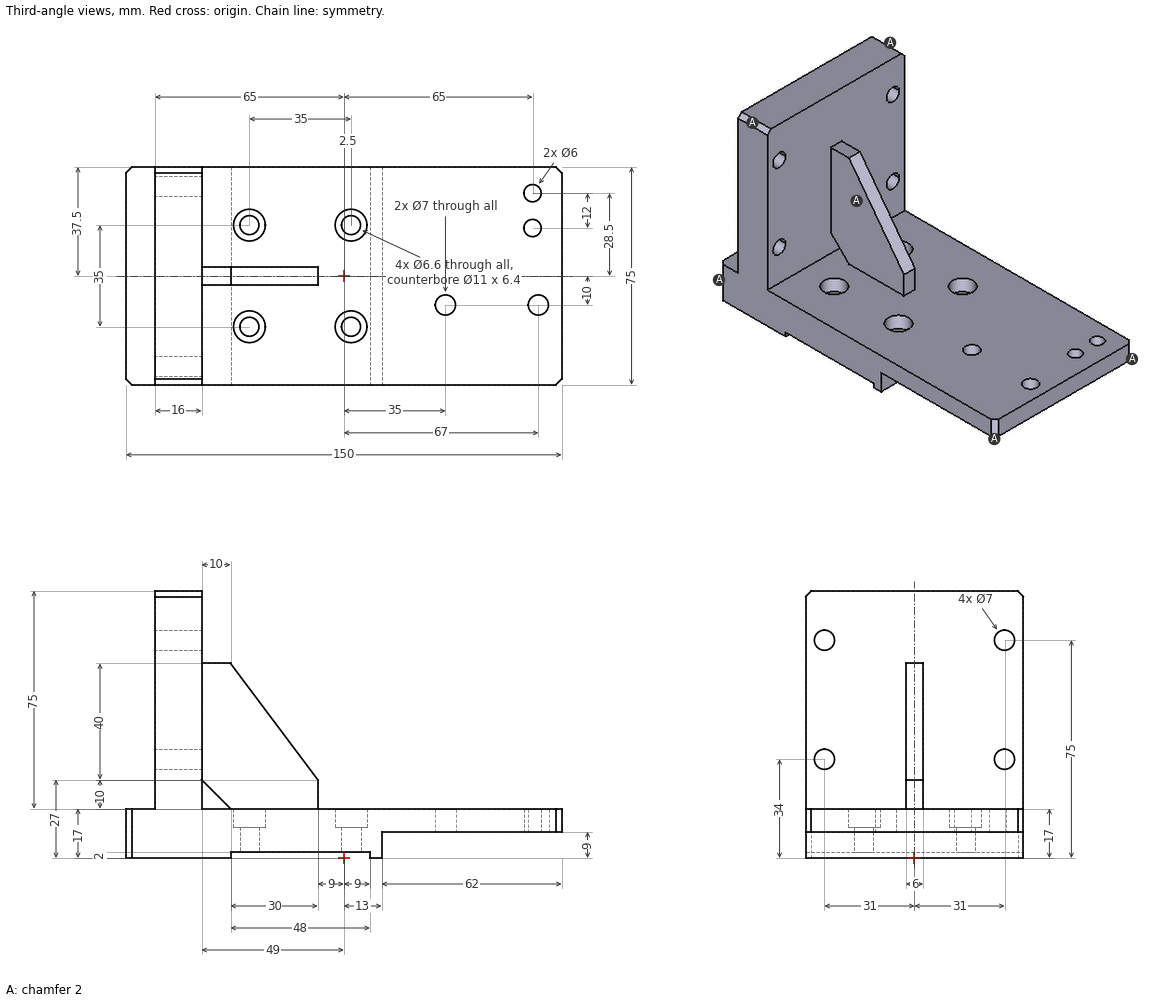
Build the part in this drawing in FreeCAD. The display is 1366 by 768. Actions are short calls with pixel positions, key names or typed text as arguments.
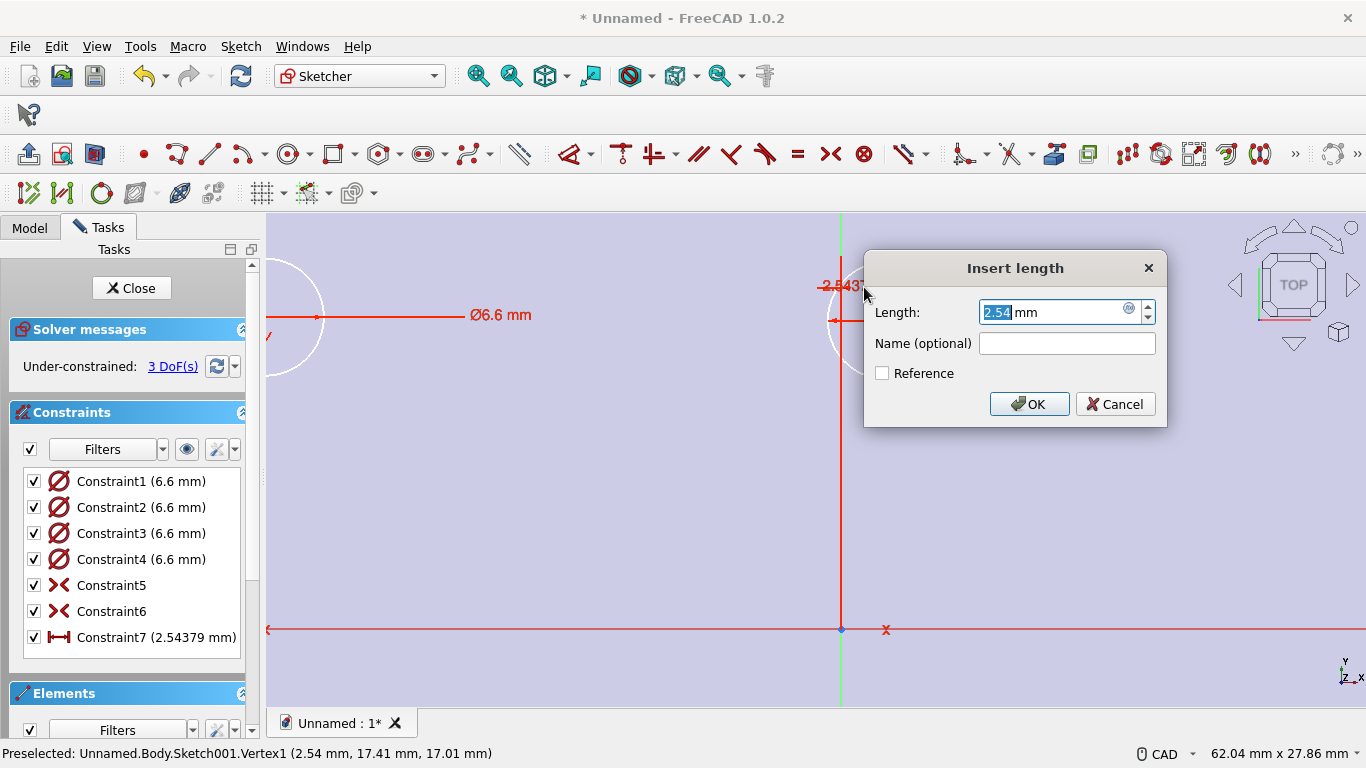
text(2.5)
key(Return)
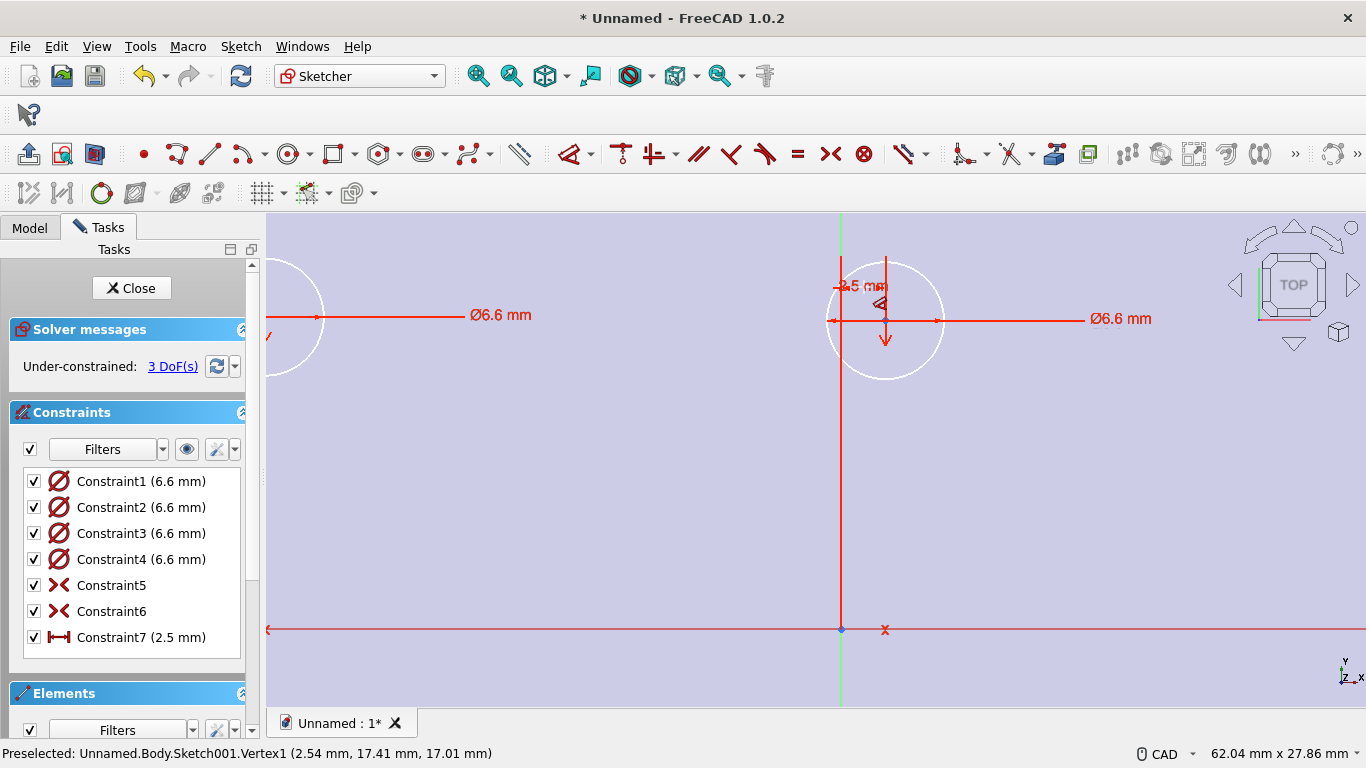
click(886, 321)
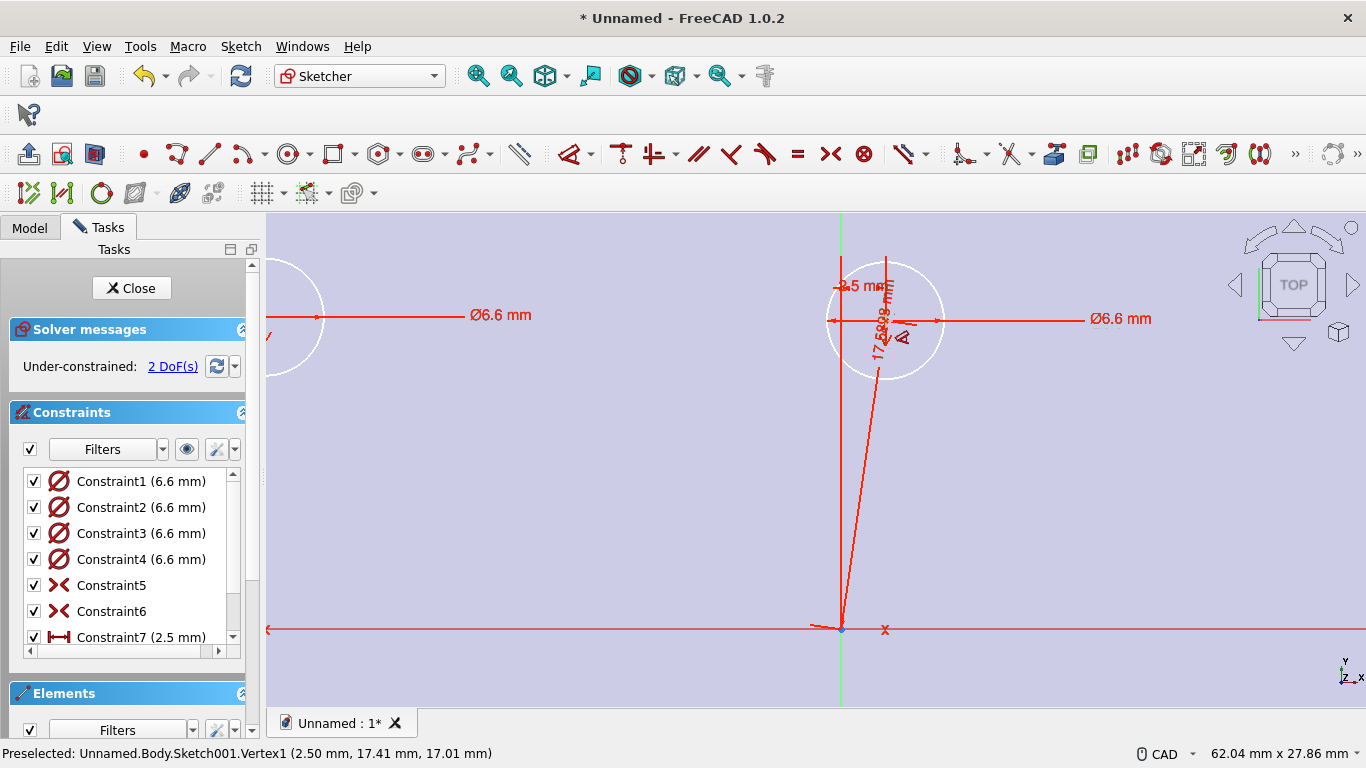
scroll(888, 322, down, 4)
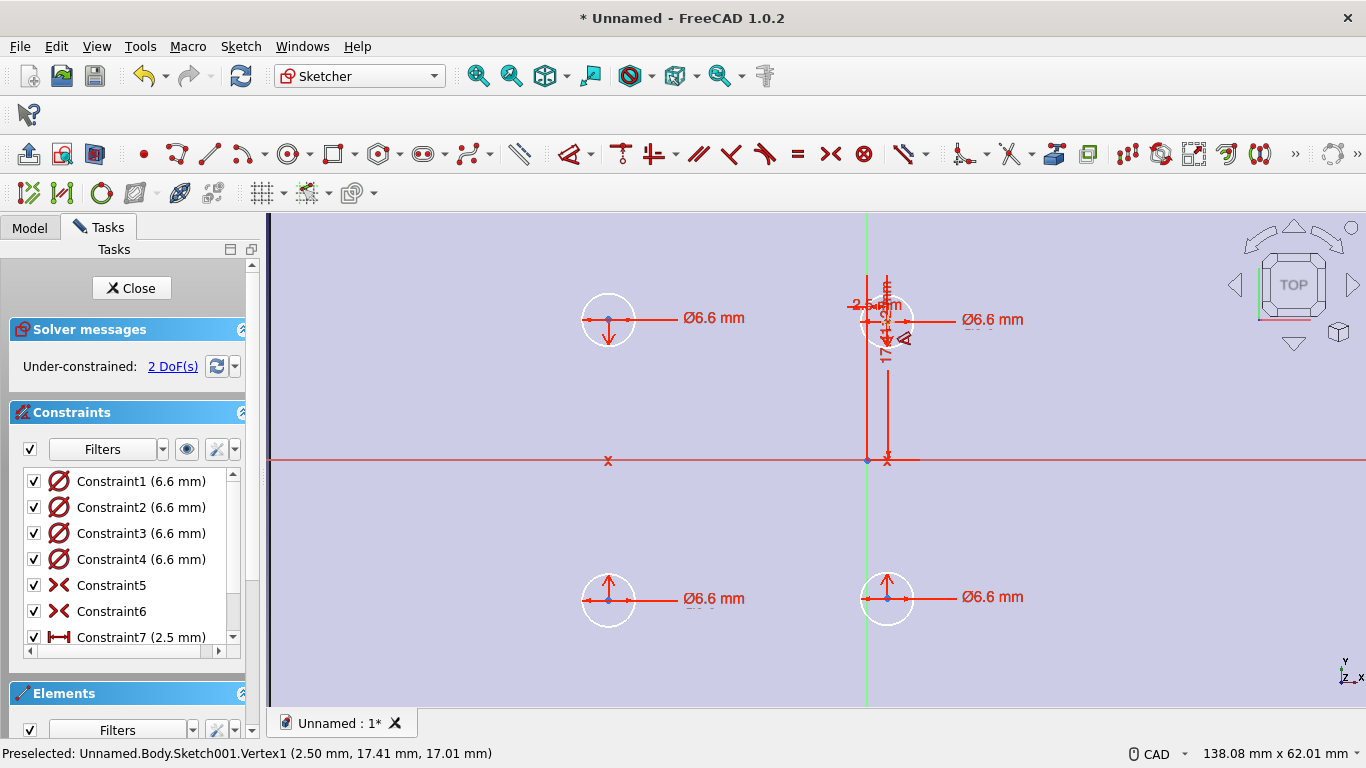
click(609, 320)
click(748, 286)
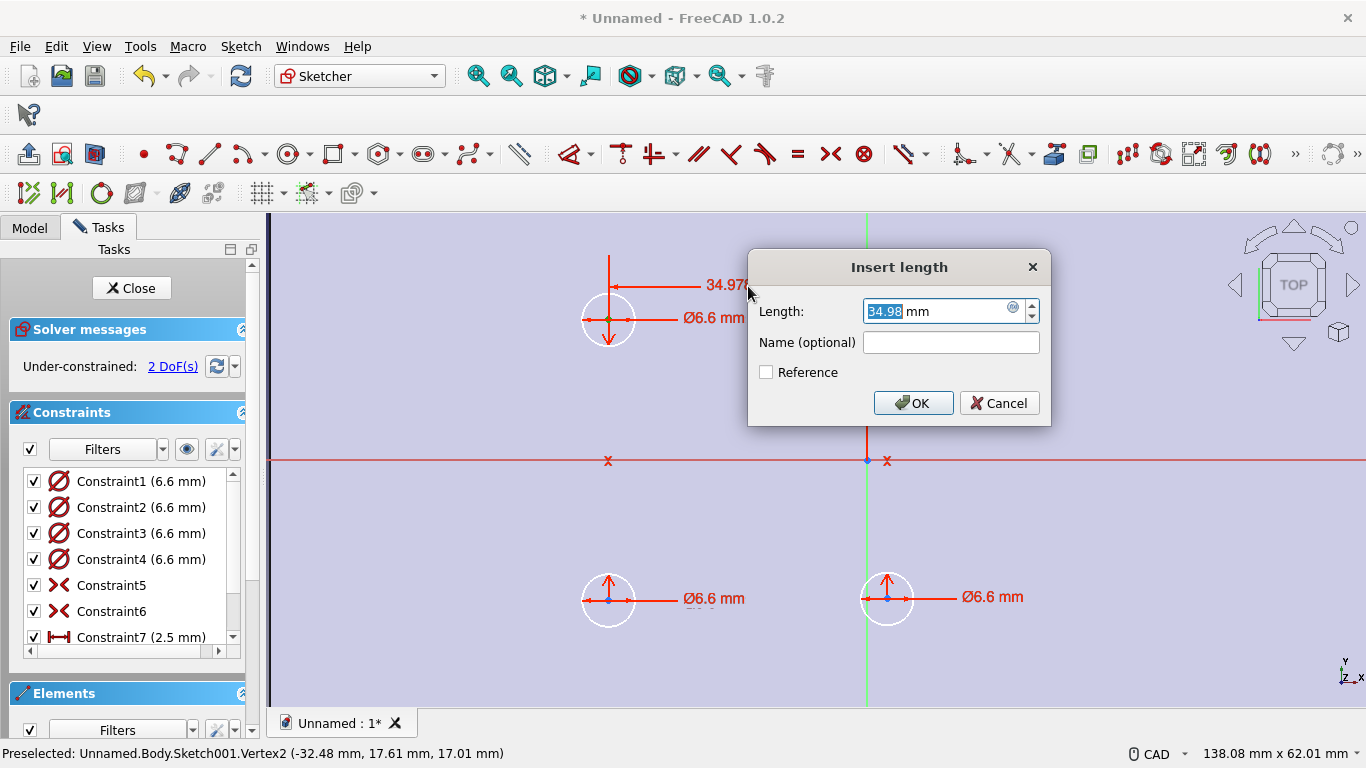
text(35)
key(Return)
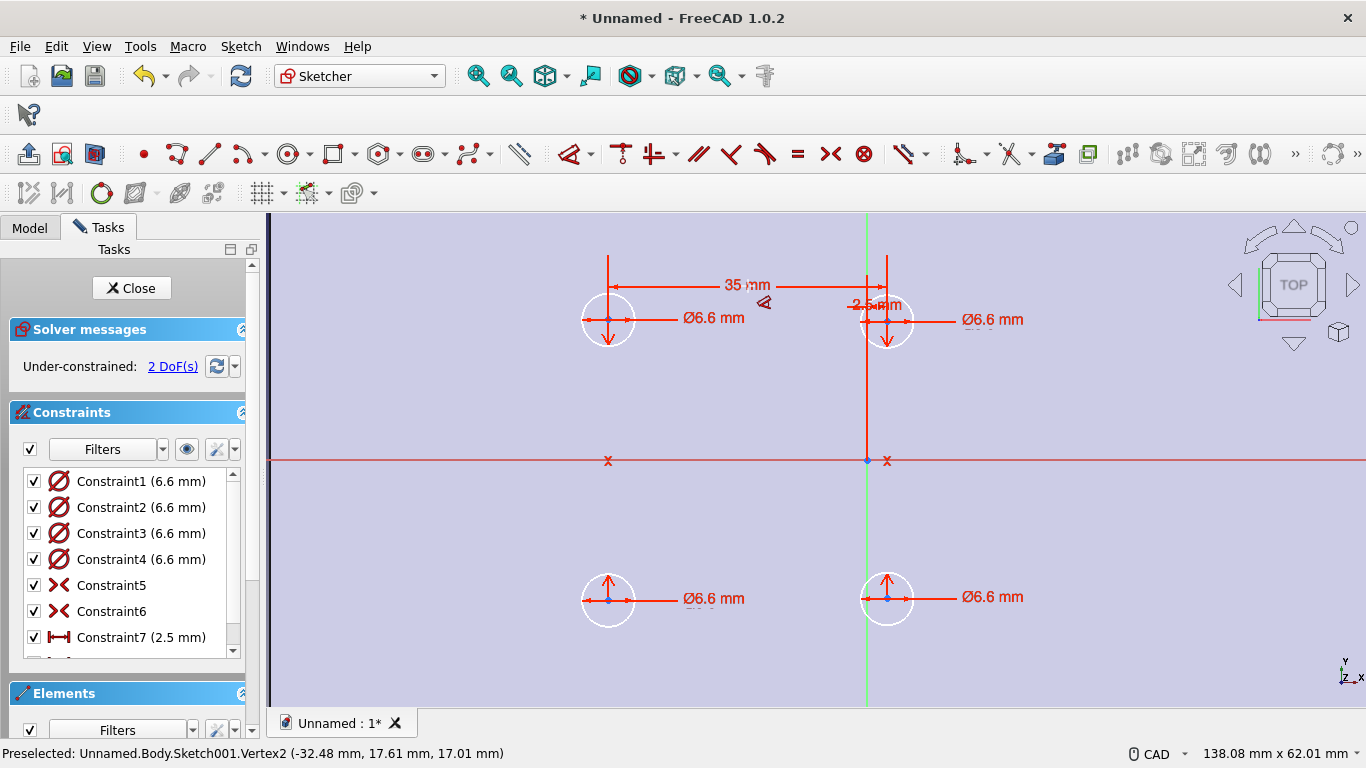
click(608, 320)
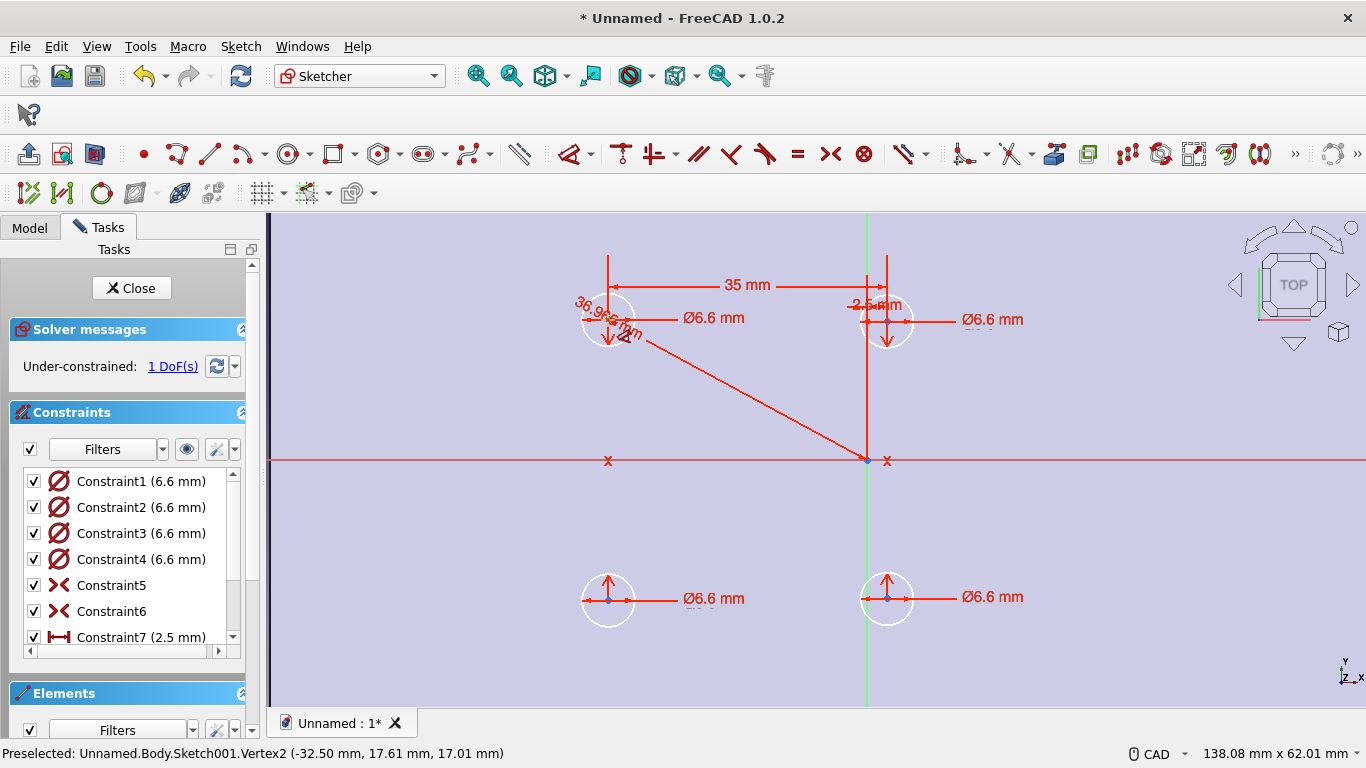
click(608, 601)
click(574, 396)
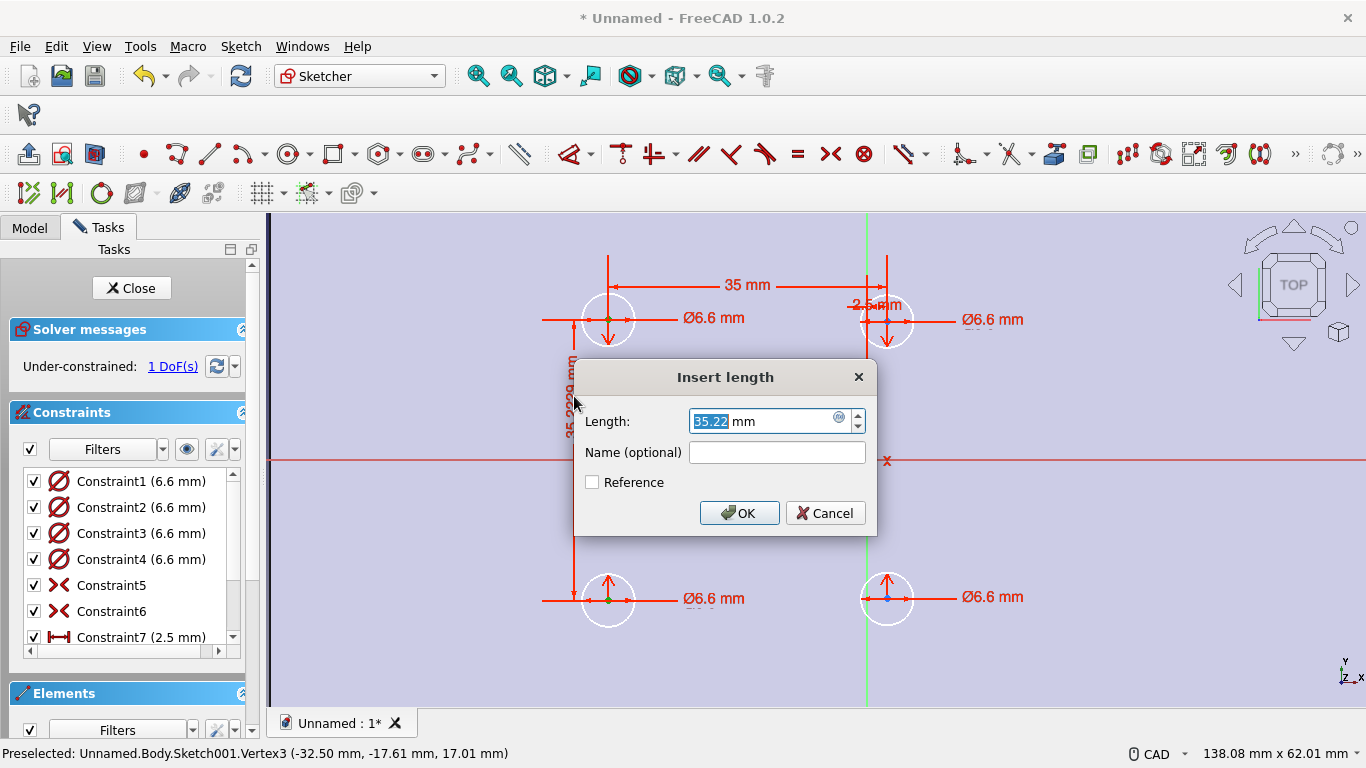
text(35)
key(Return)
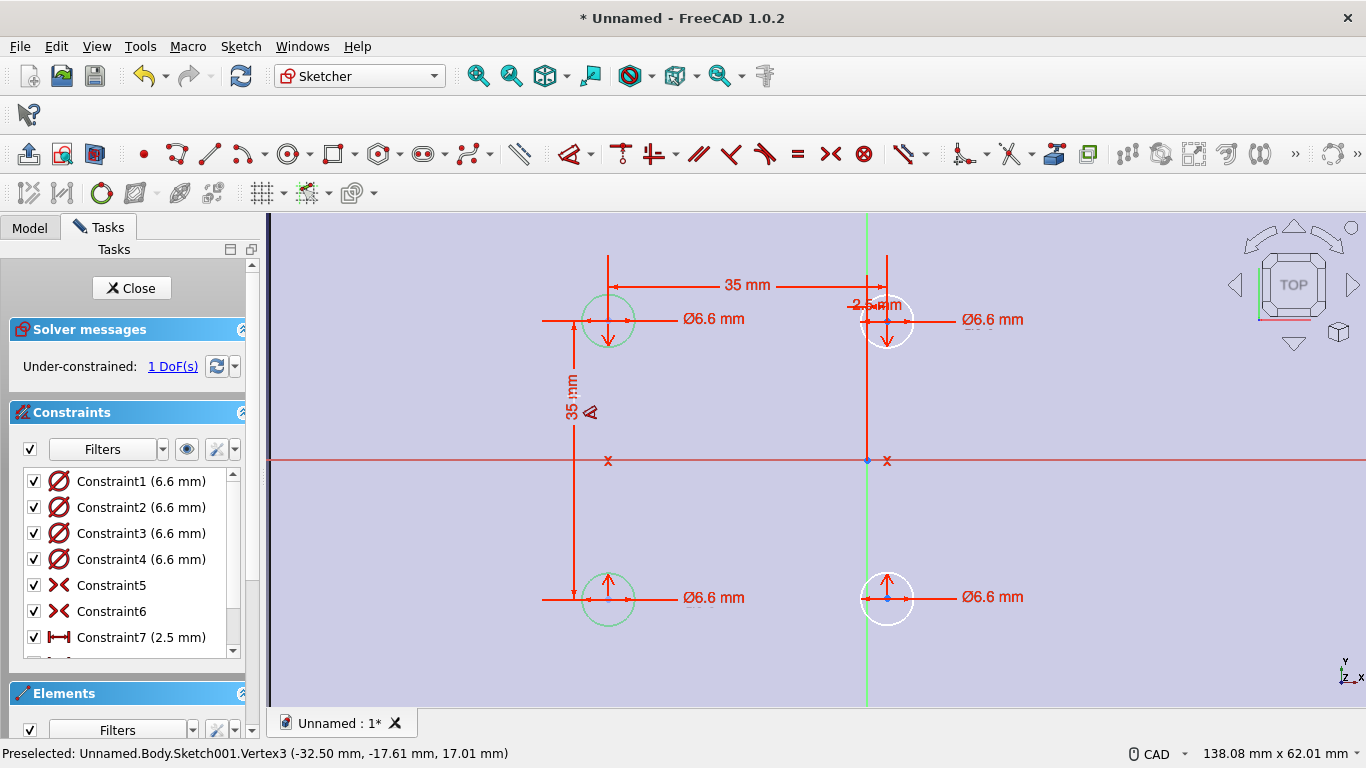
click(887, 322)